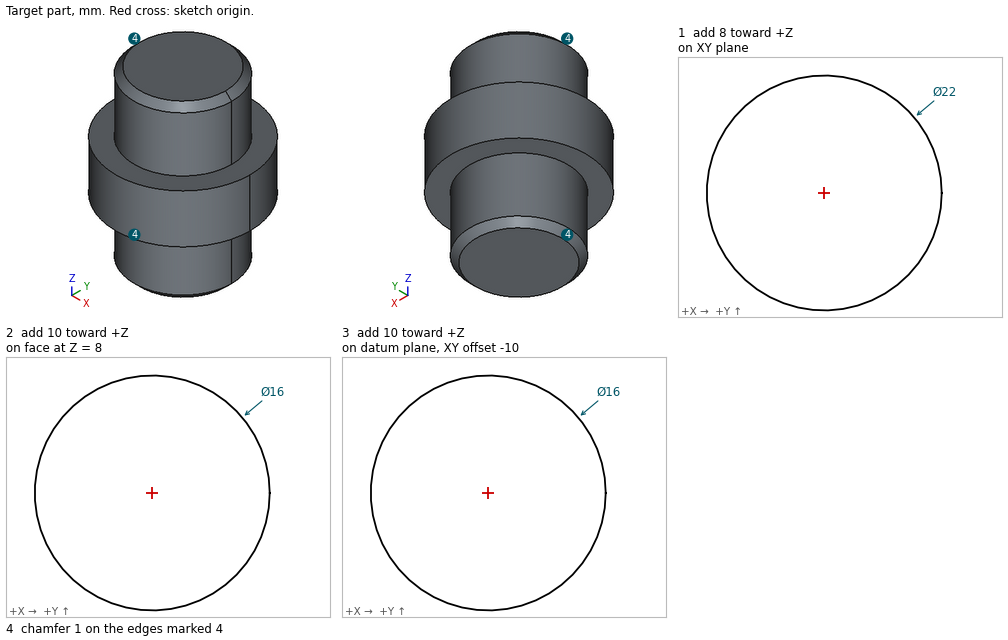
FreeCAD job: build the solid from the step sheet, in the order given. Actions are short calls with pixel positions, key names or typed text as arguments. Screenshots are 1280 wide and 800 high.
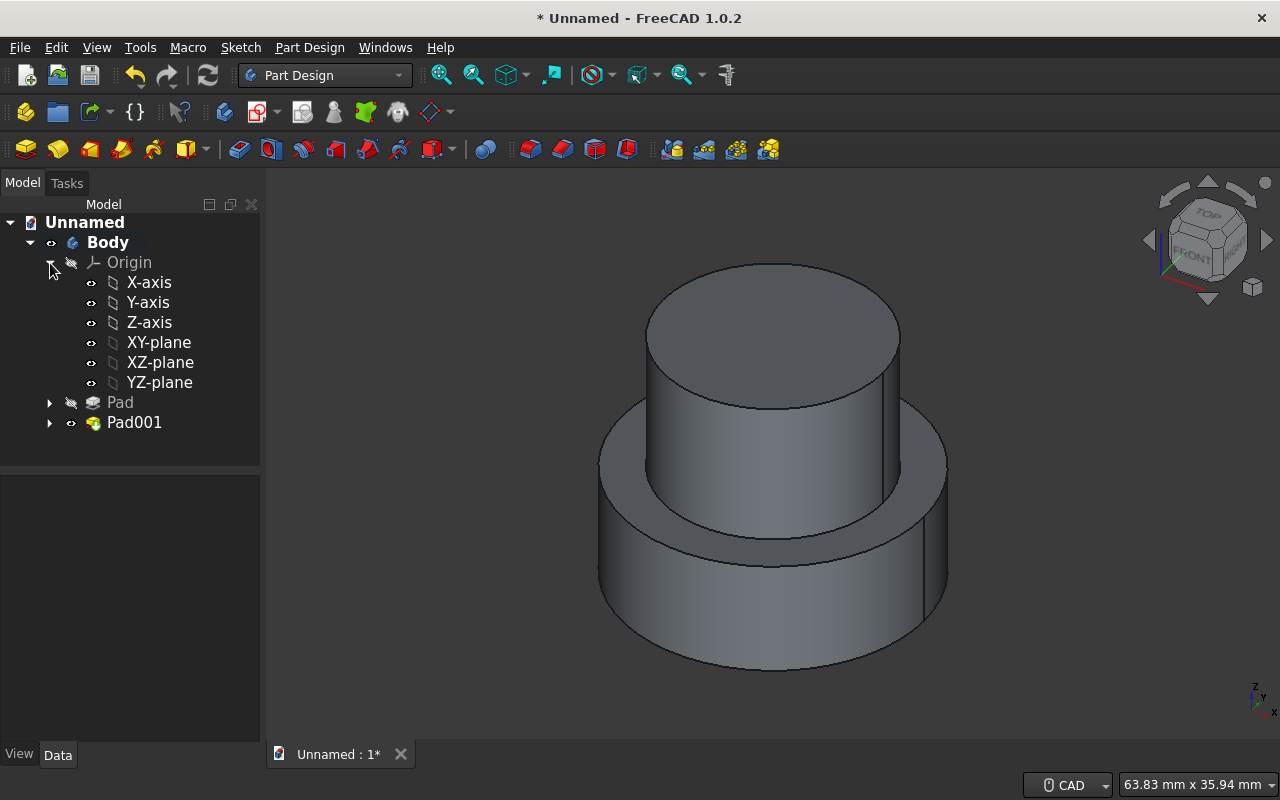
click(136, 343)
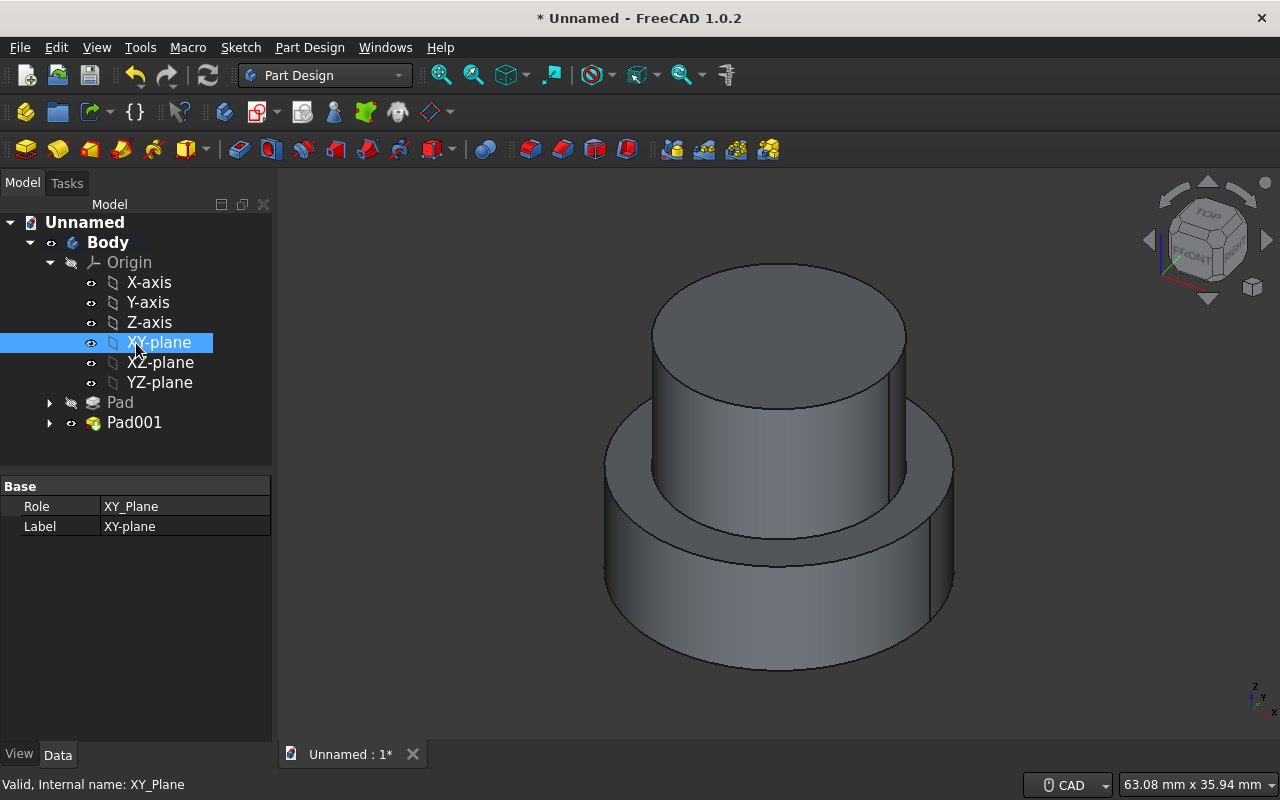
click(430, 112)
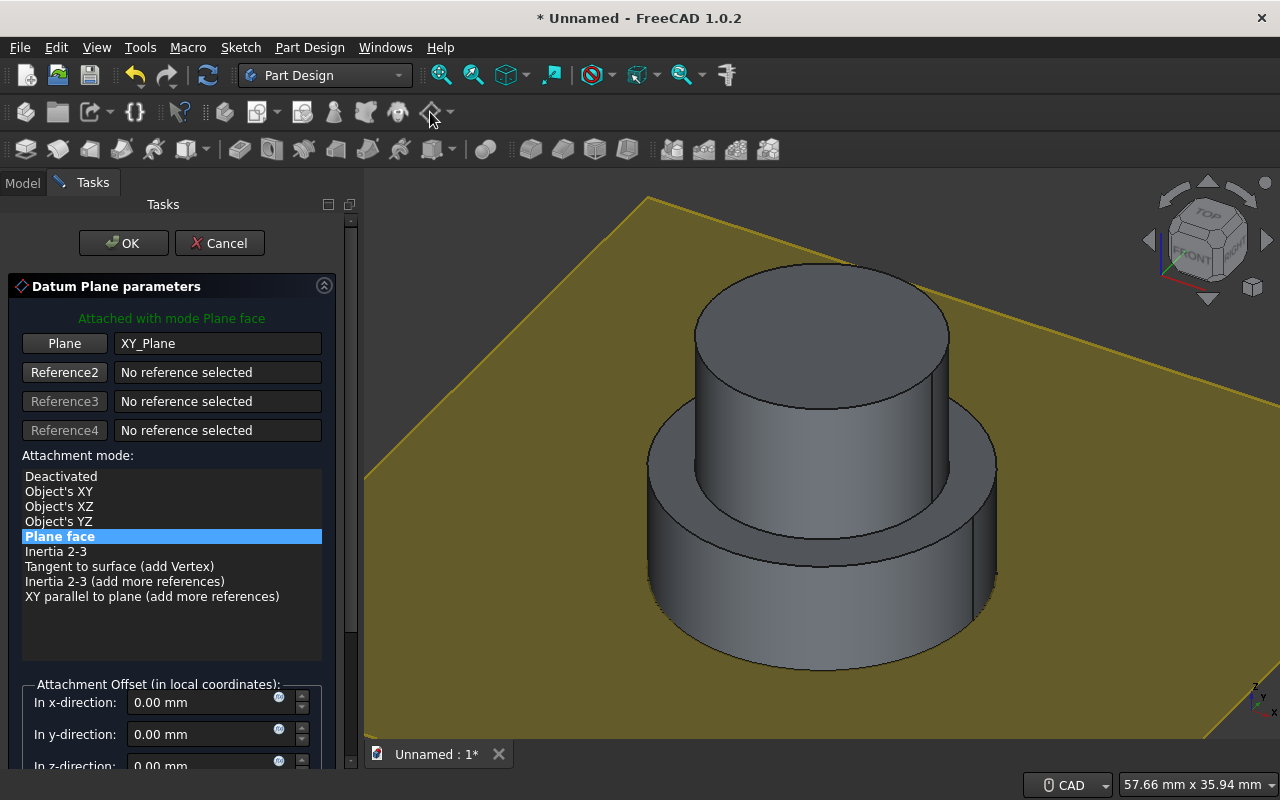
scroll(351, 491, down, 2)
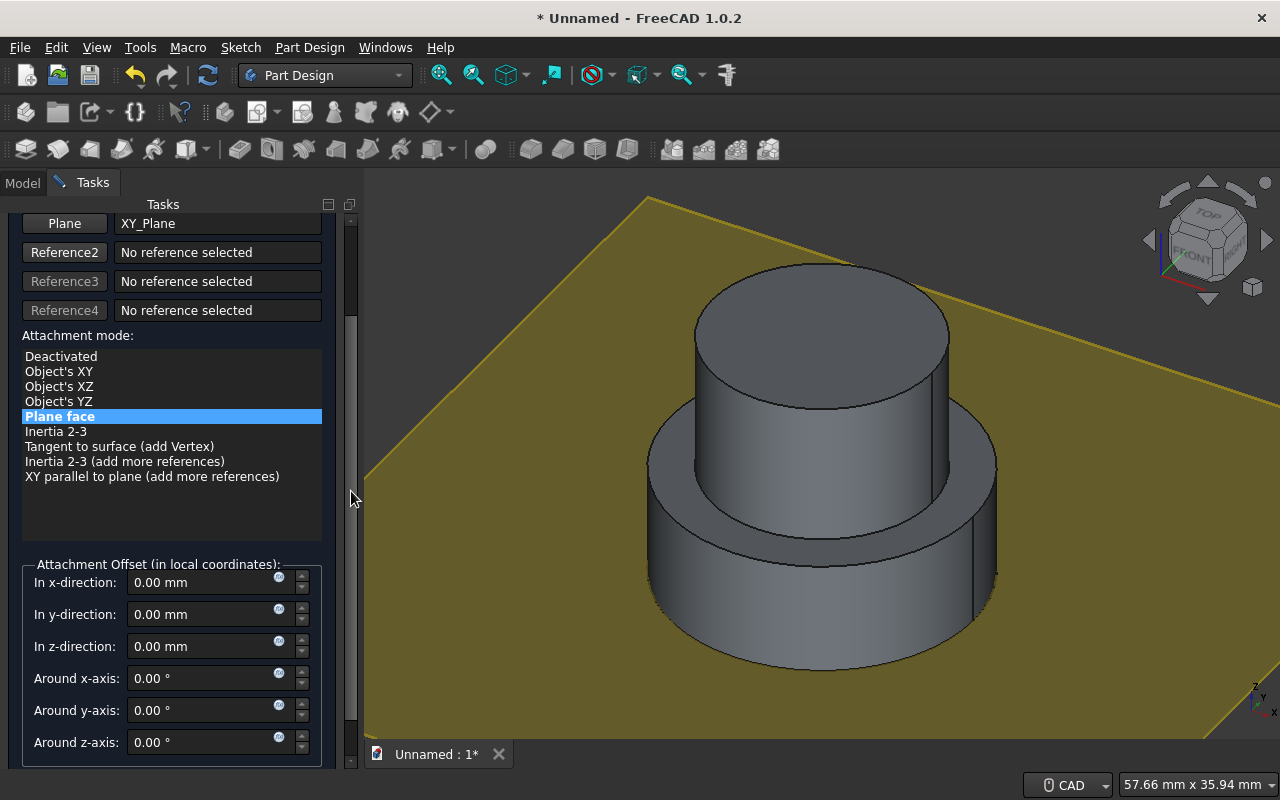
triple_click(210, 646)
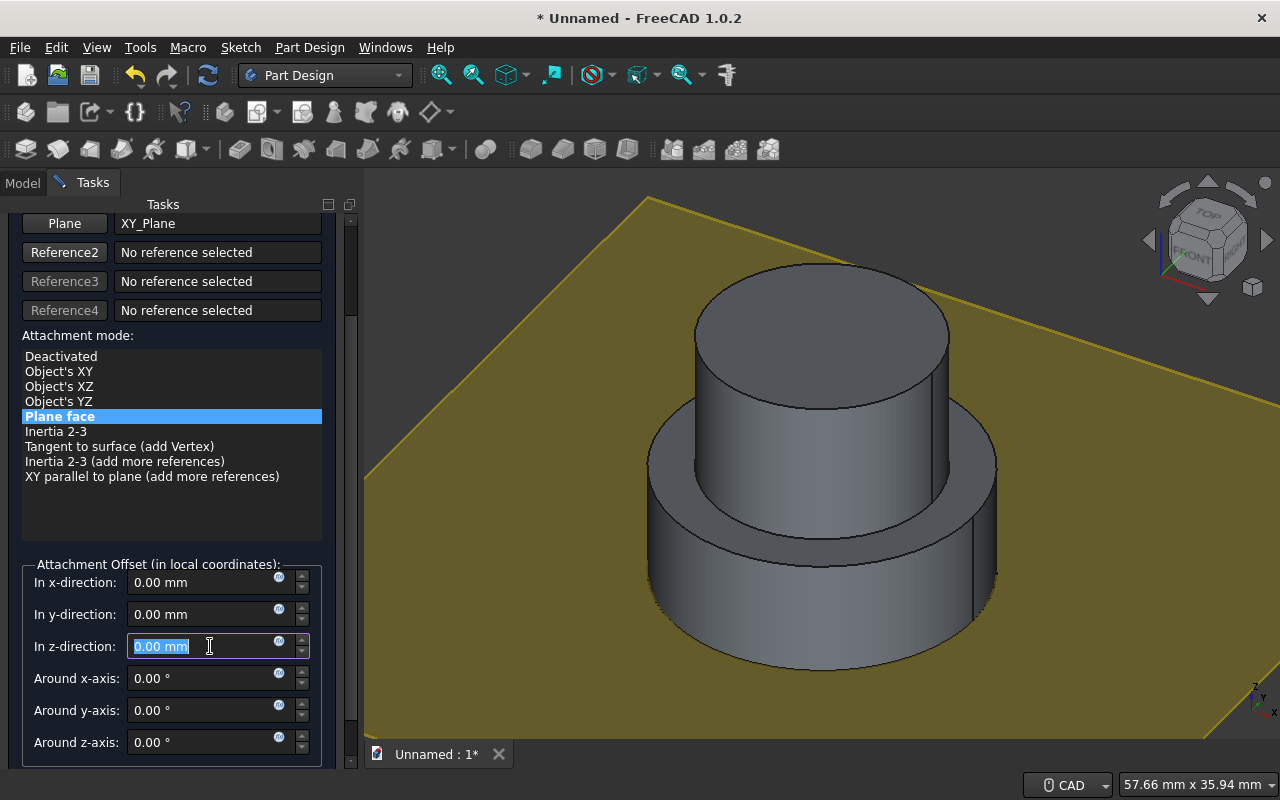
text(-10)
key(Tab)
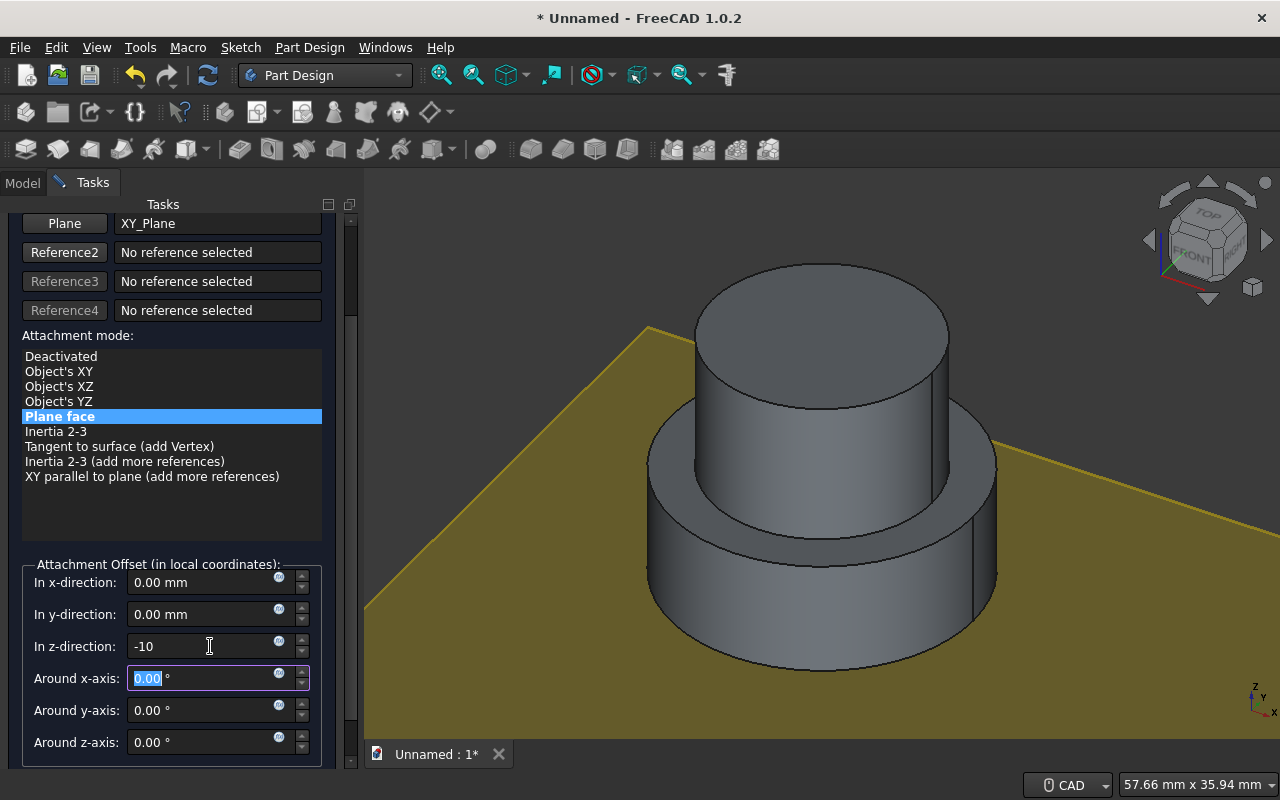
scroll(351, 491, up, 3)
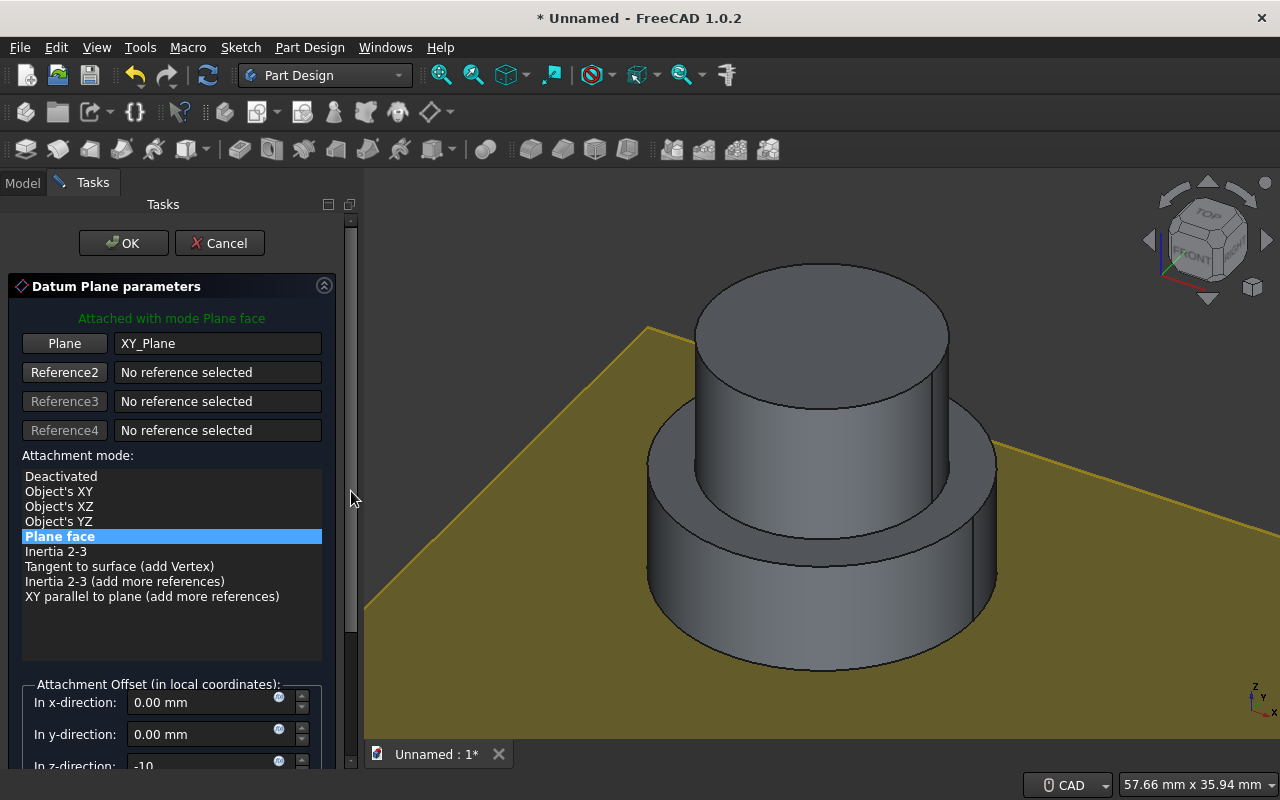
click(124, 243)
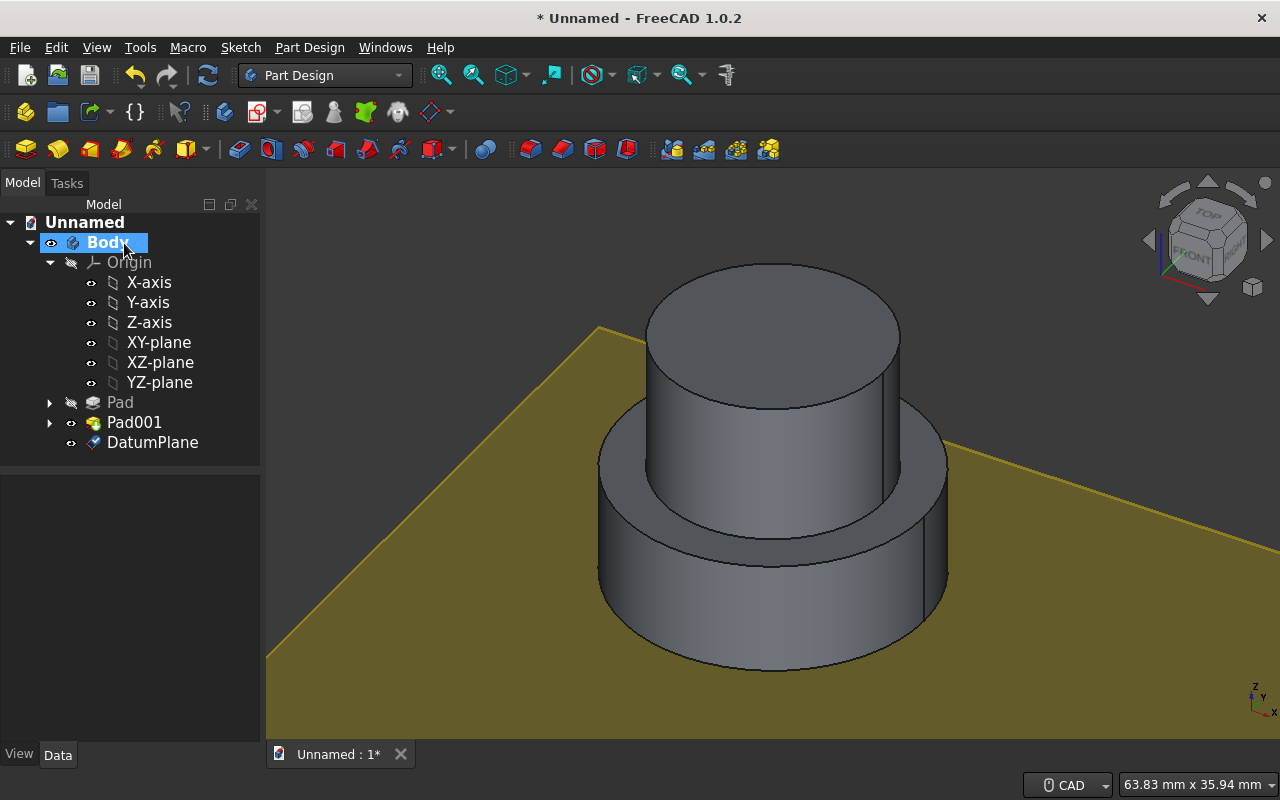
click(116, 443)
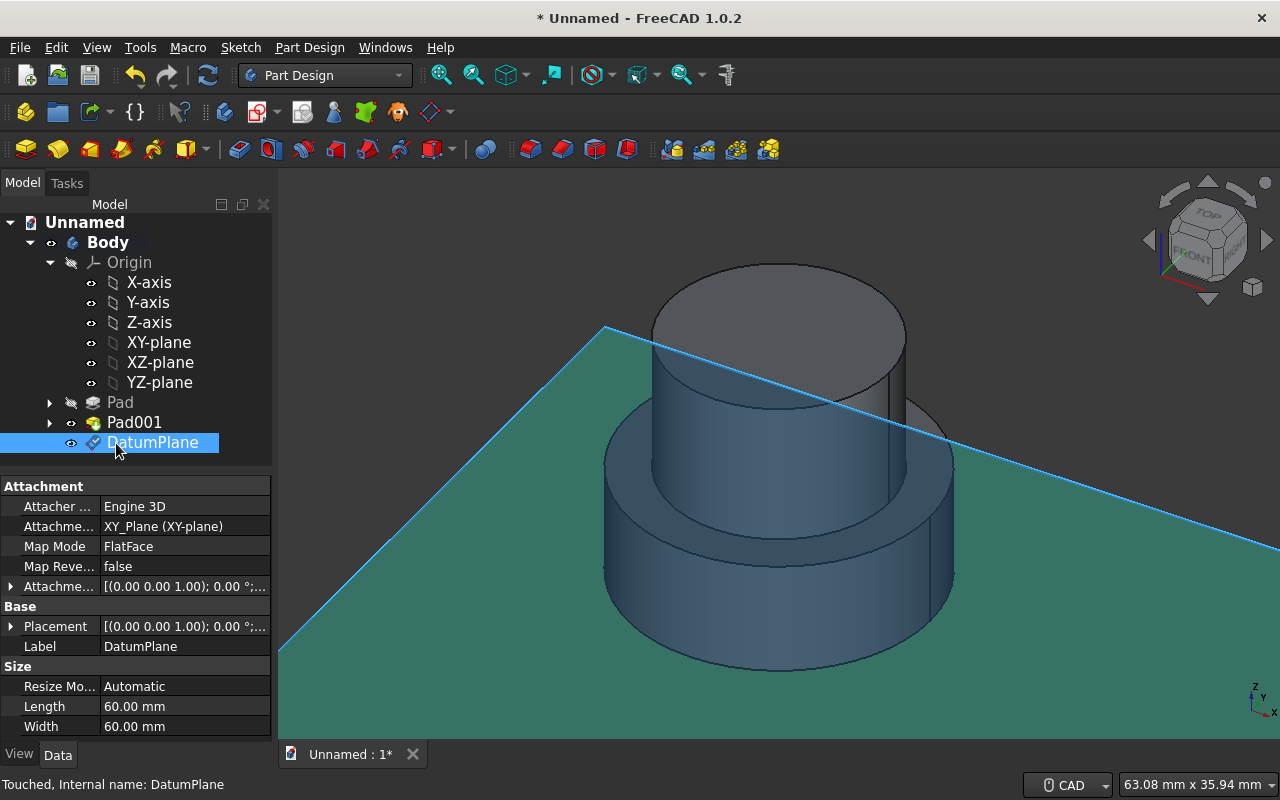
click(258, 112)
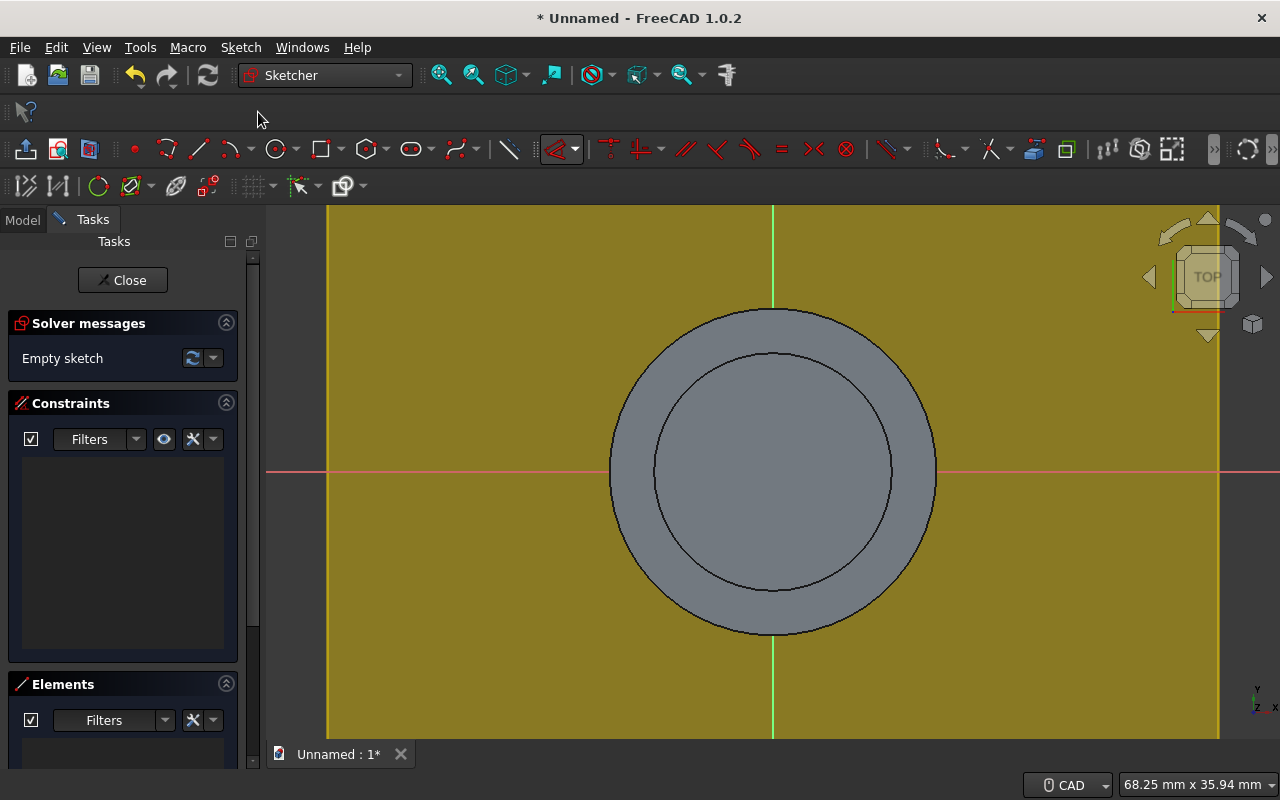
key(q)
key(s)